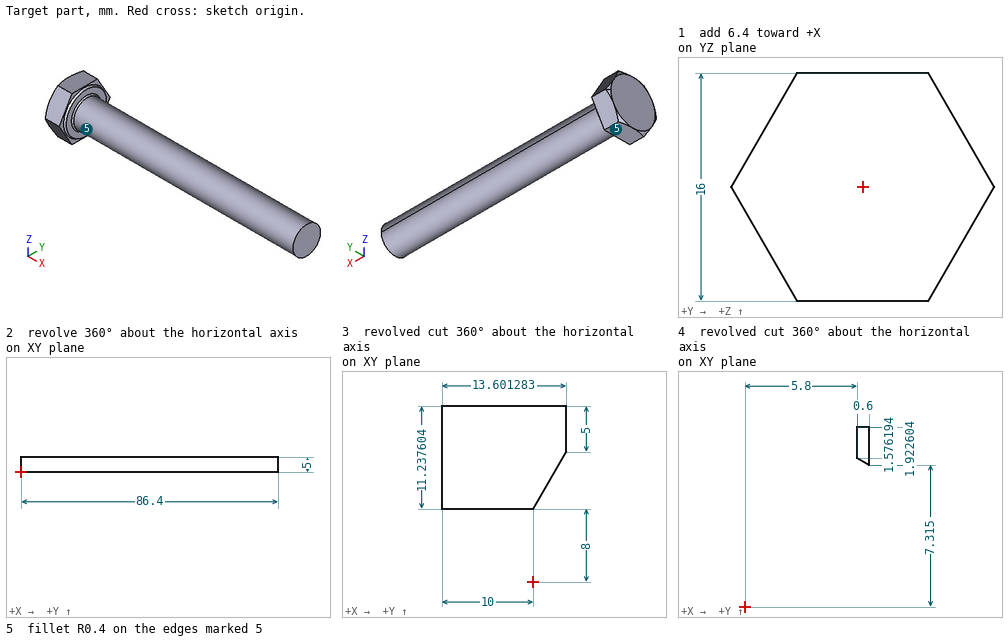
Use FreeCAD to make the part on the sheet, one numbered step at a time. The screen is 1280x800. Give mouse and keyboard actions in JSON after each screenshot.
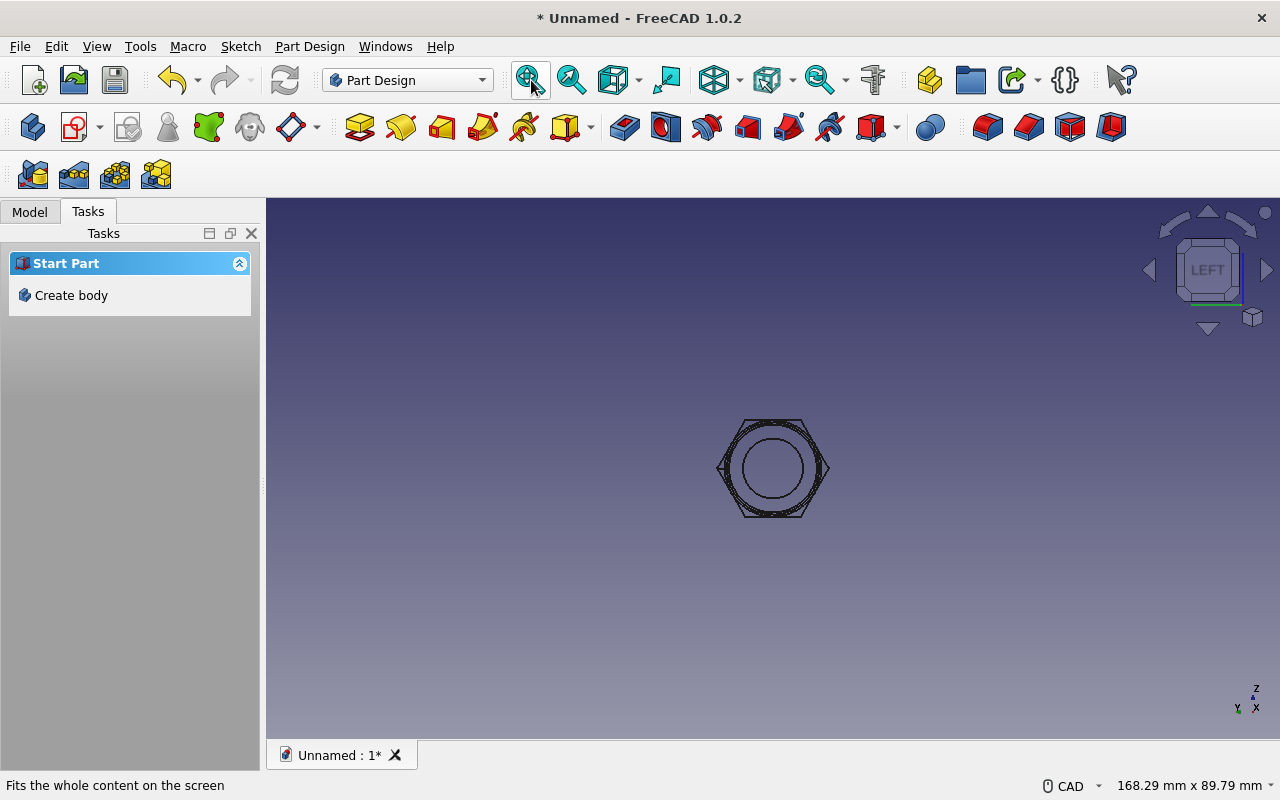
{"action": "key", "text": "0"}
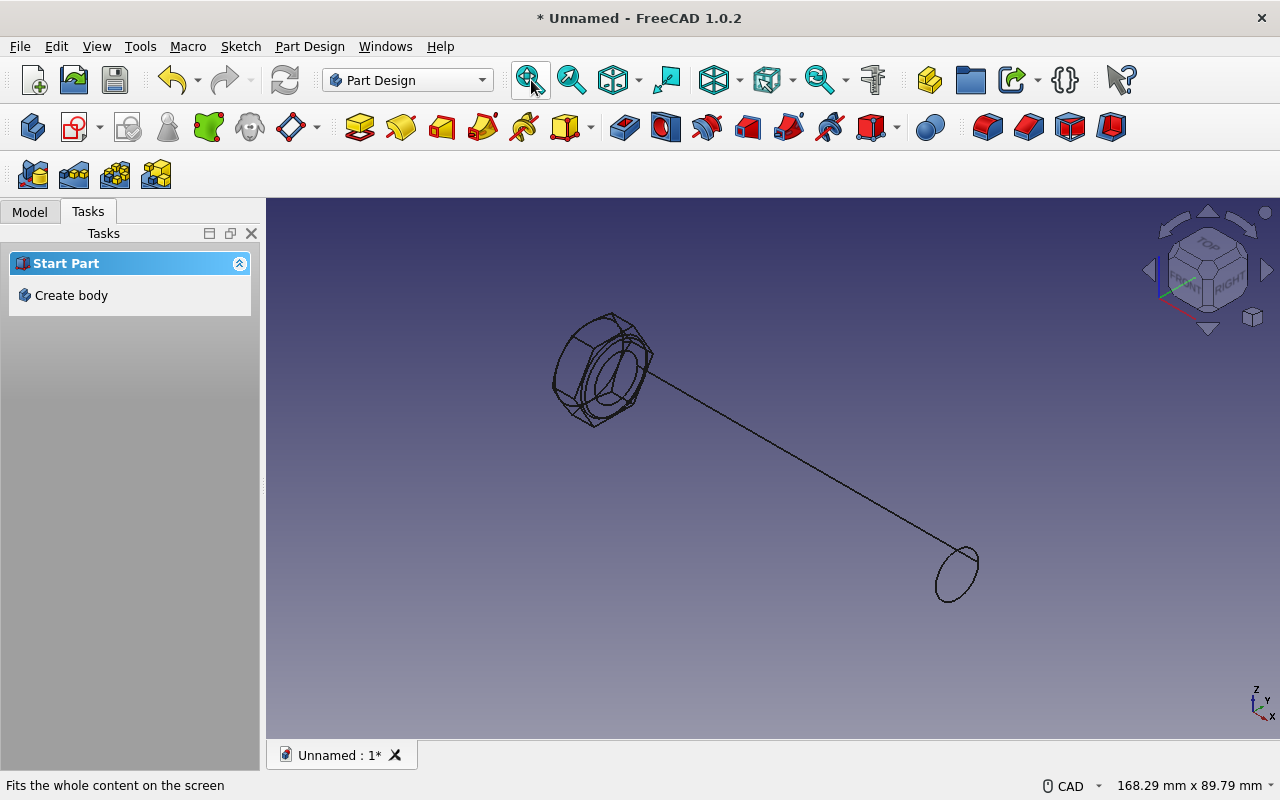
{"action": "left_click", "coordinate": [595, 389]}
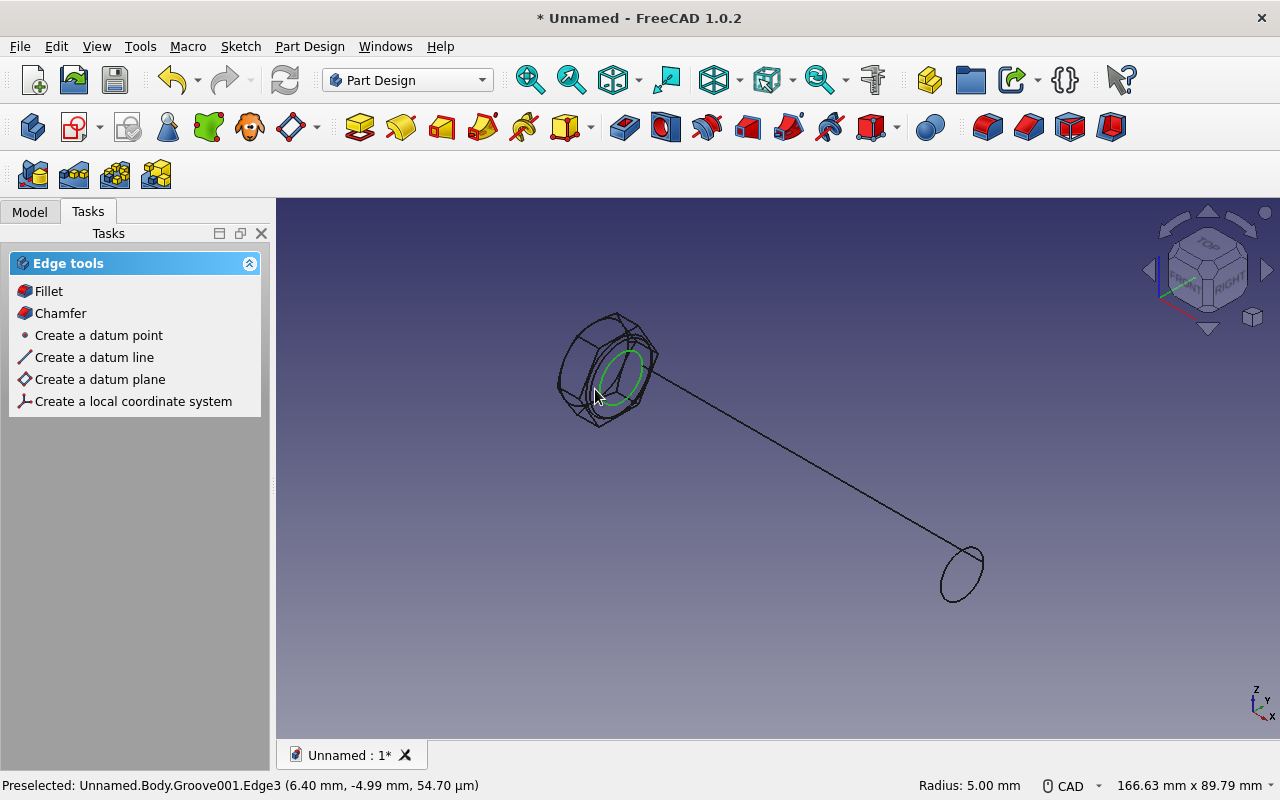
{"action": "key", "text": "v 1"}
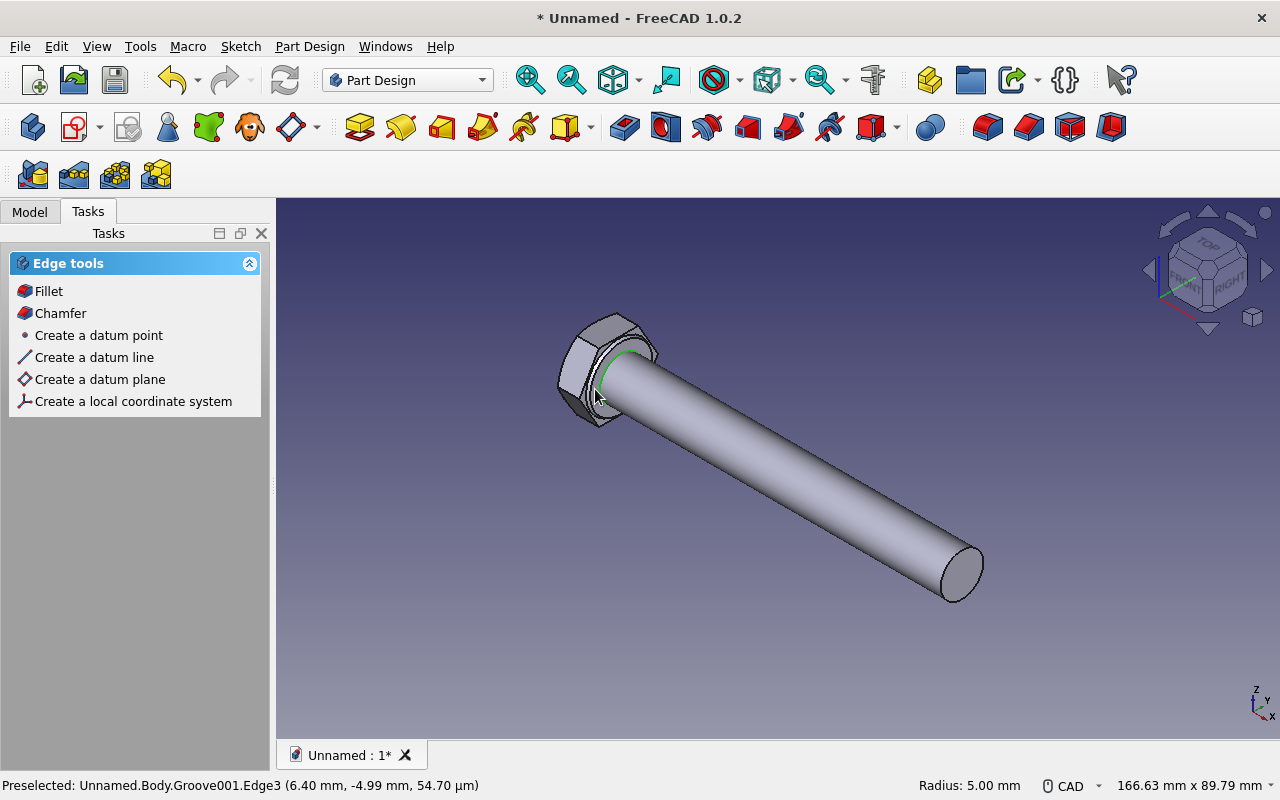
{"action": "left_click", "coordinate": [988, 128]}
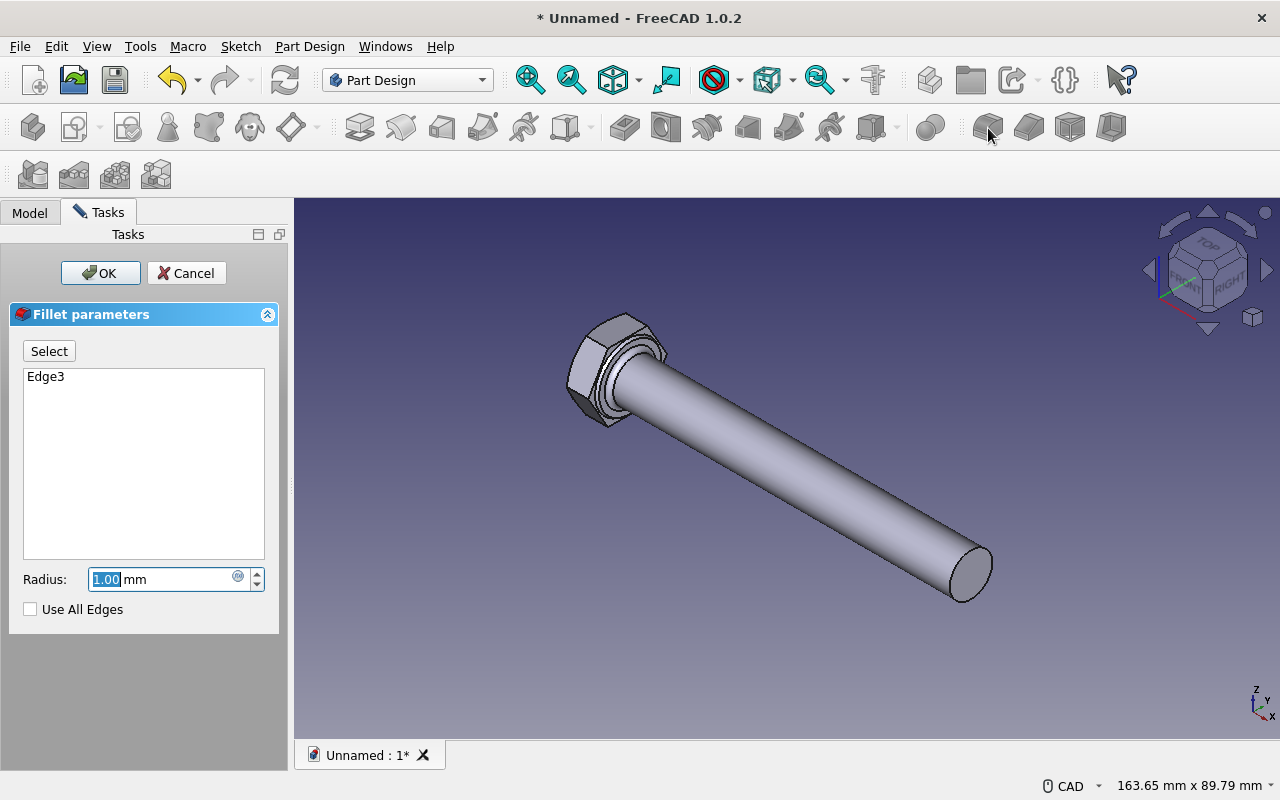
{"action": "type", "text": "0.4"}
{"action": "key", "text": "Tab"}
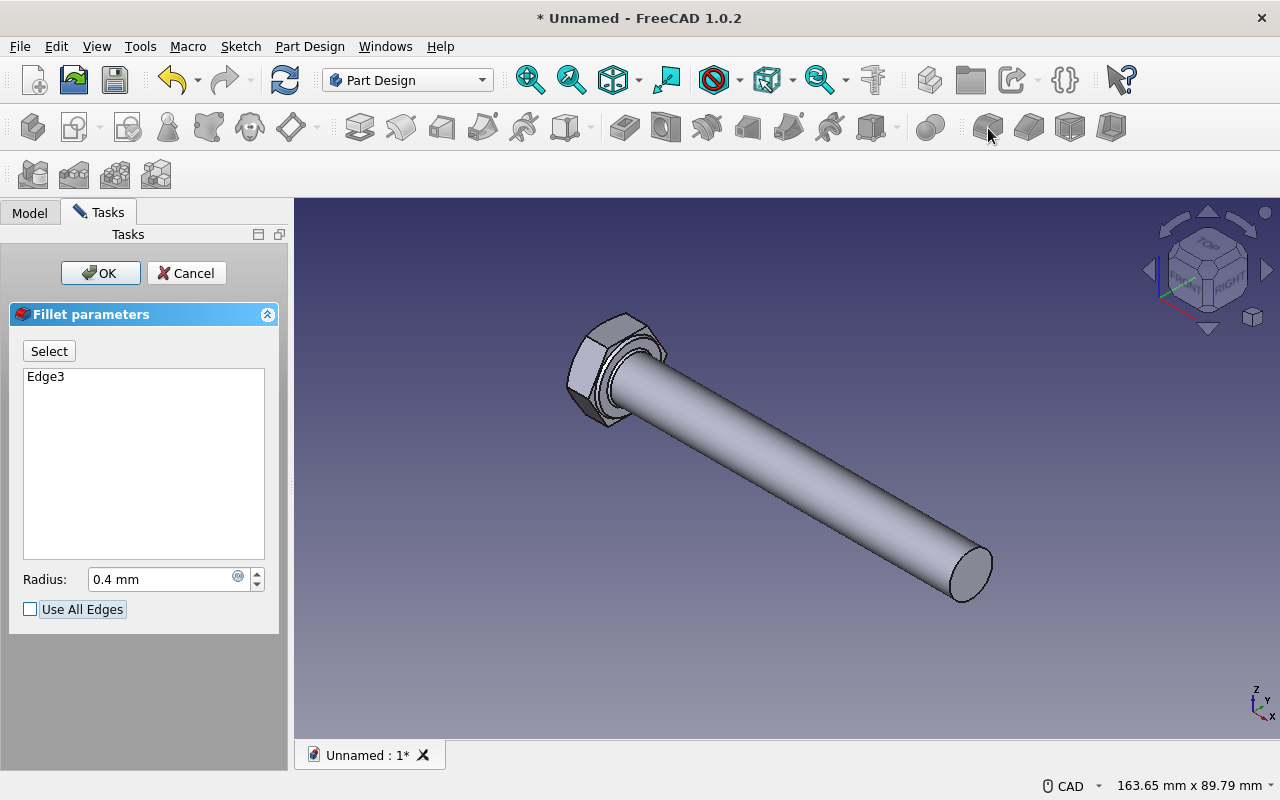
{"action": "left_click", "coordinate": [101, 273]}